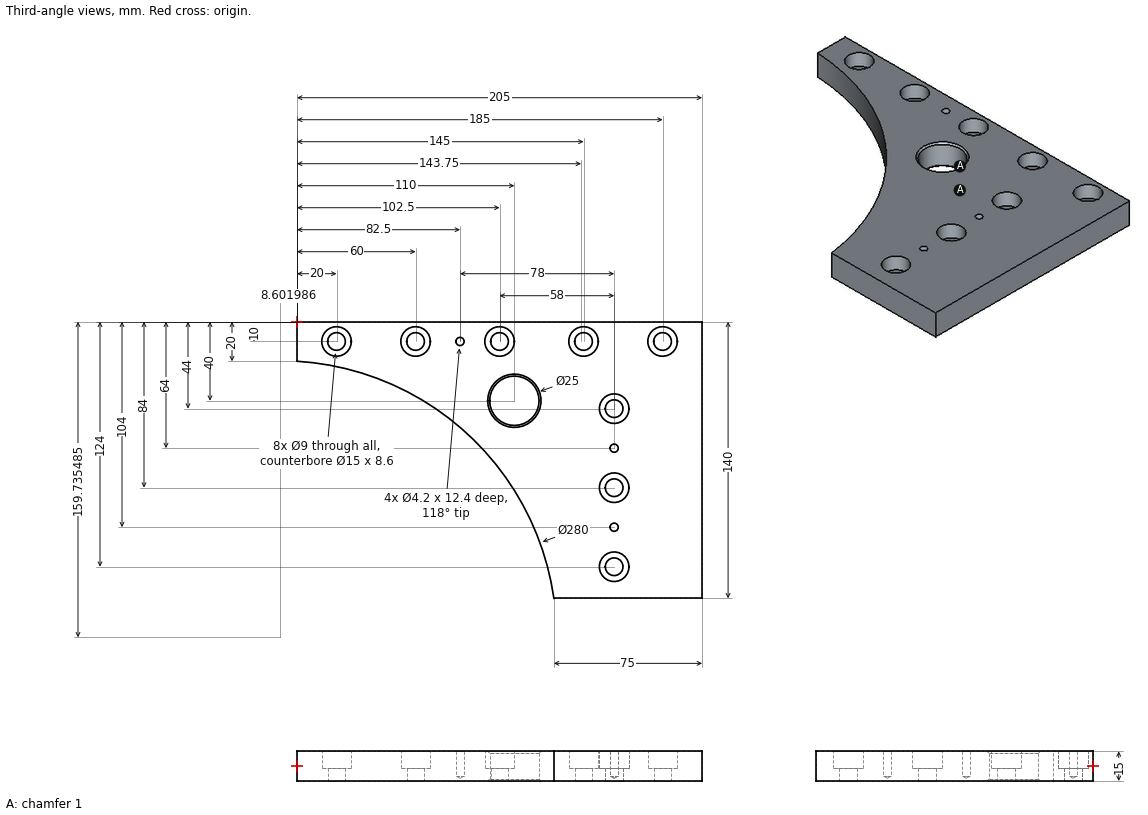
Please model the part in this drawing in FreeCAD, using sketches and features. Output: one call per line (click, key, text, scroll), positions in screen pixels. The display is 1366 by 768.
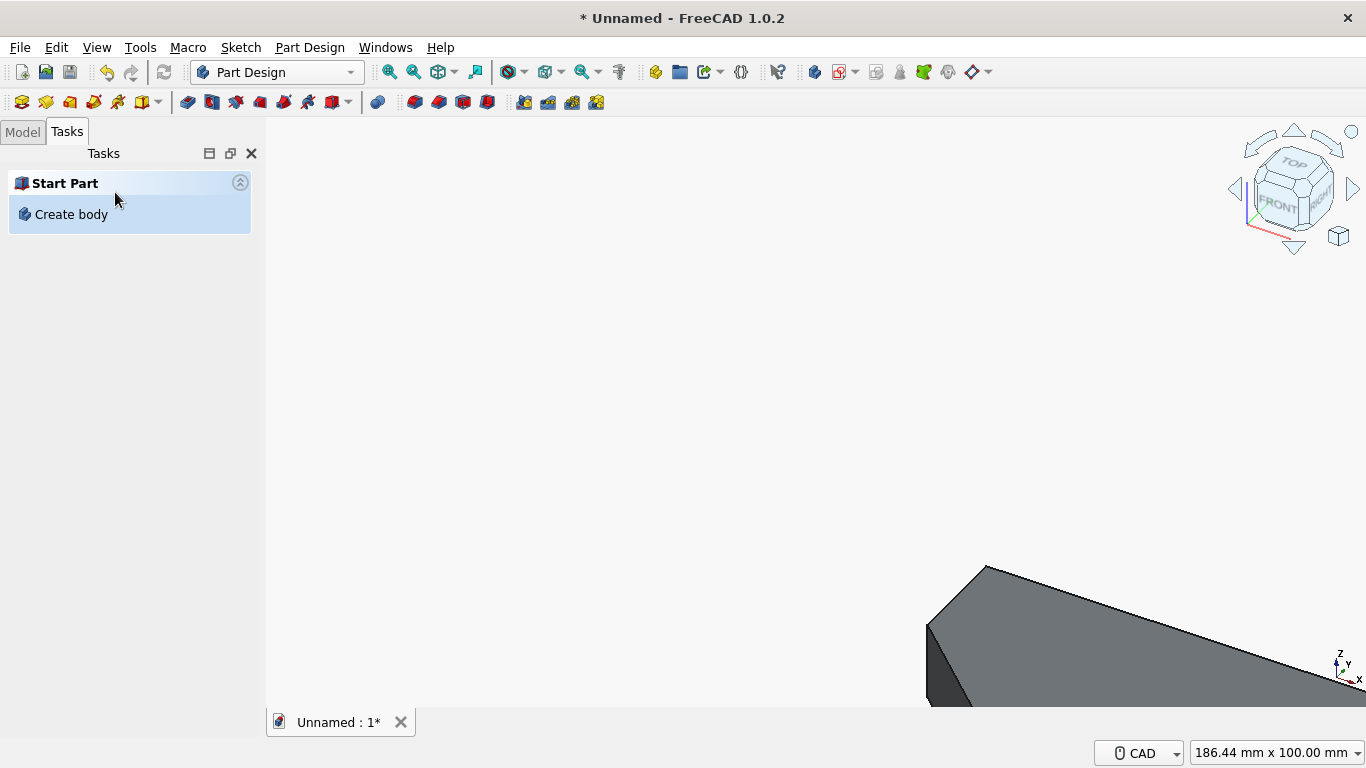
click(390, 72)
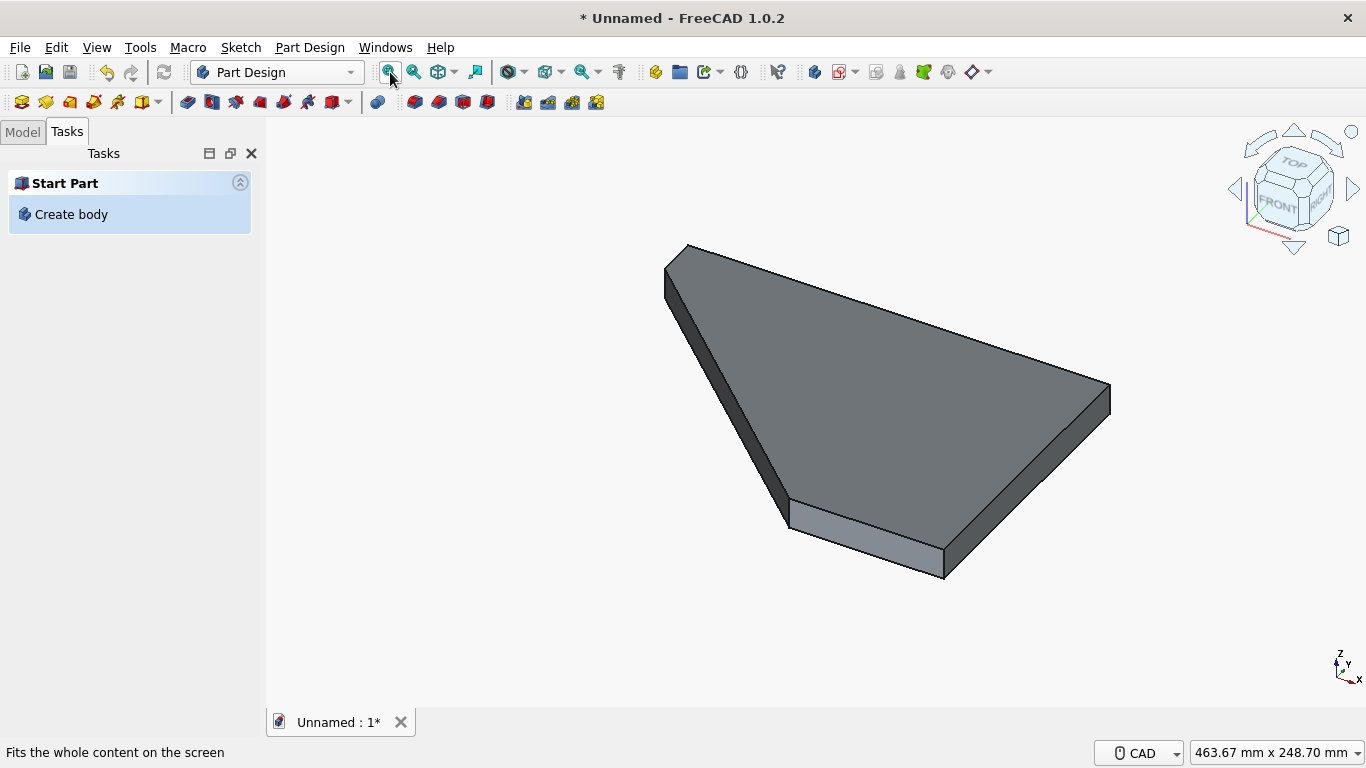
click(876, 416)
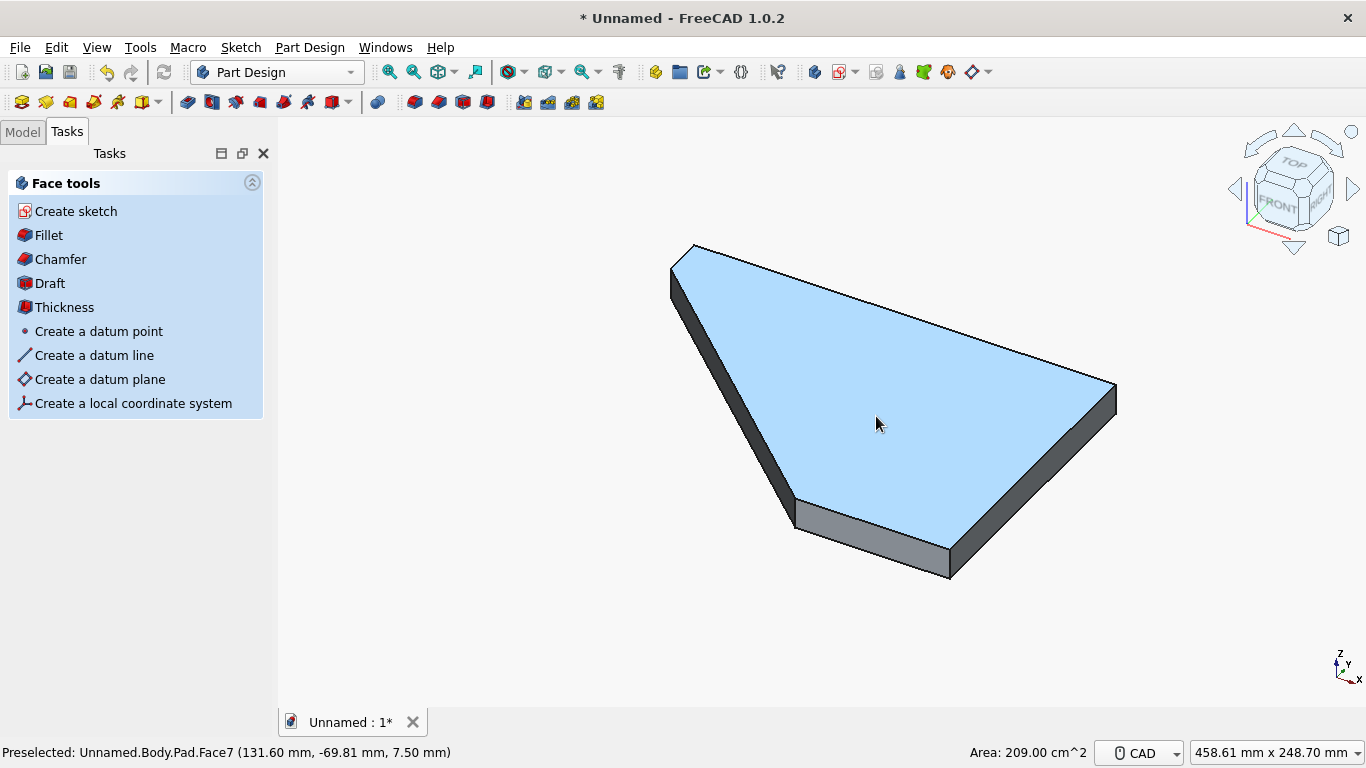
click(840, 72)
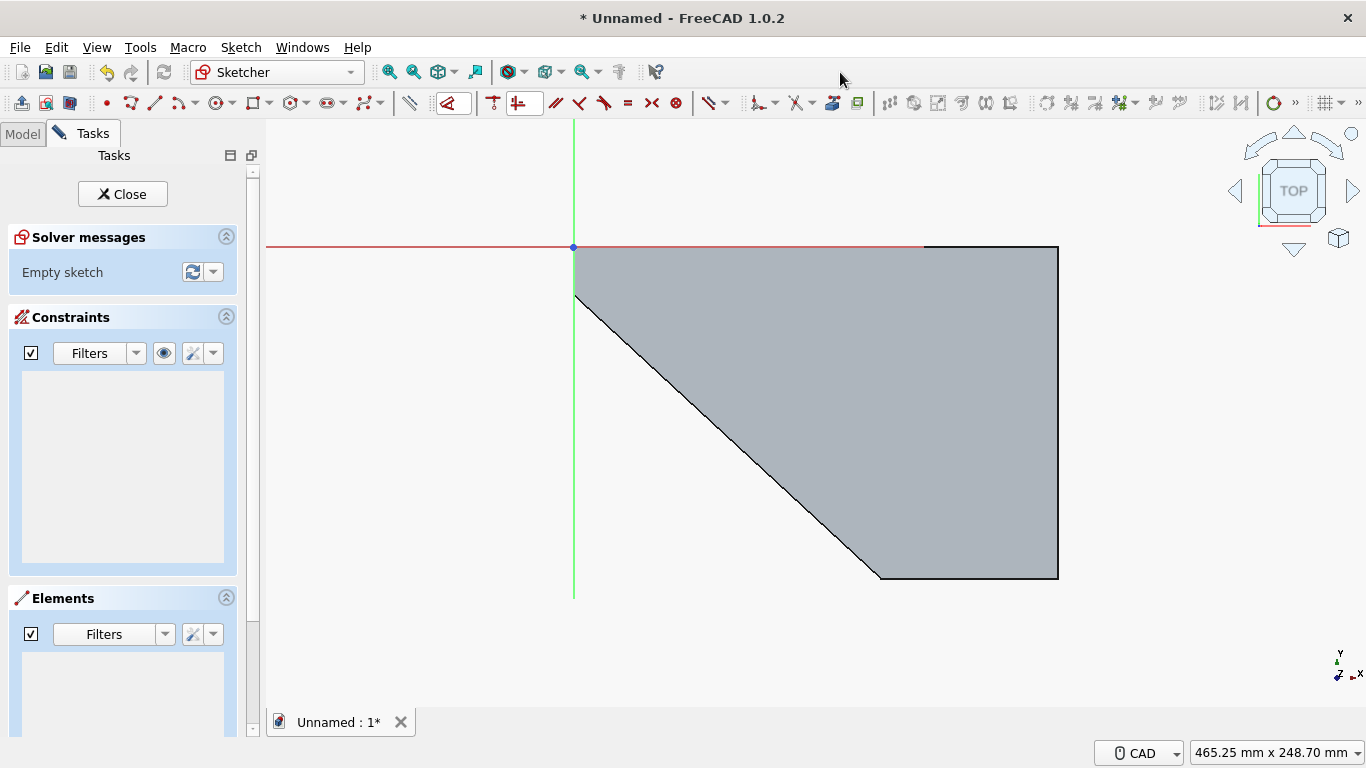
click(216, 104)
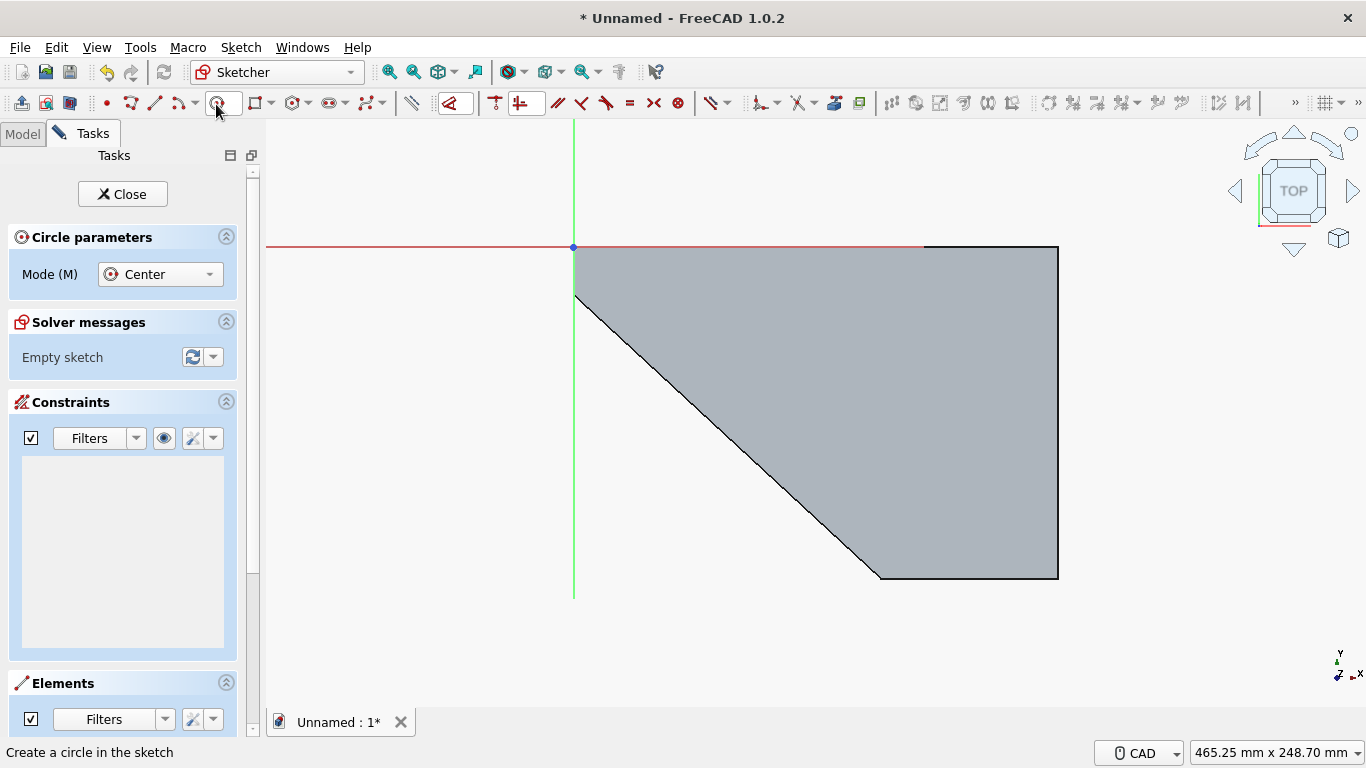
scroll(621, 271, up, 4)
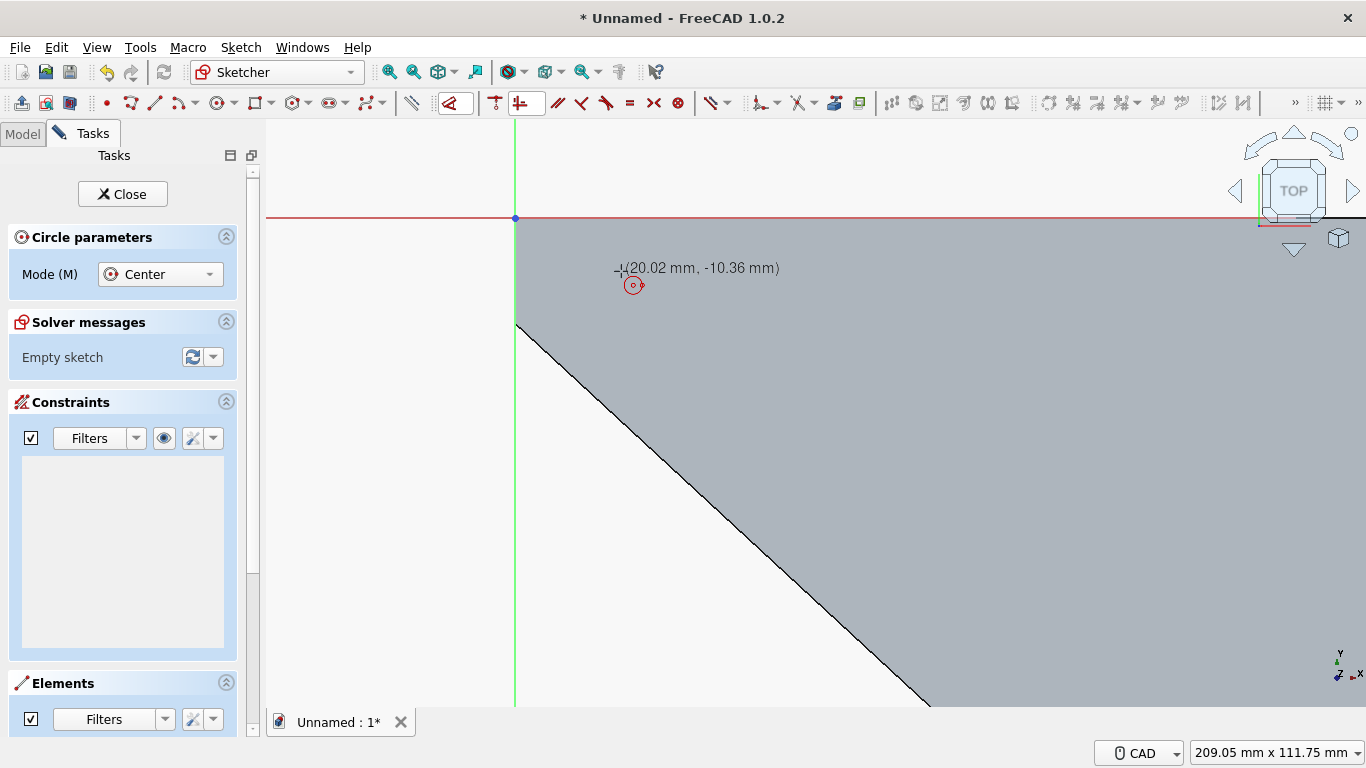
click(620, 271)
click(637, 254)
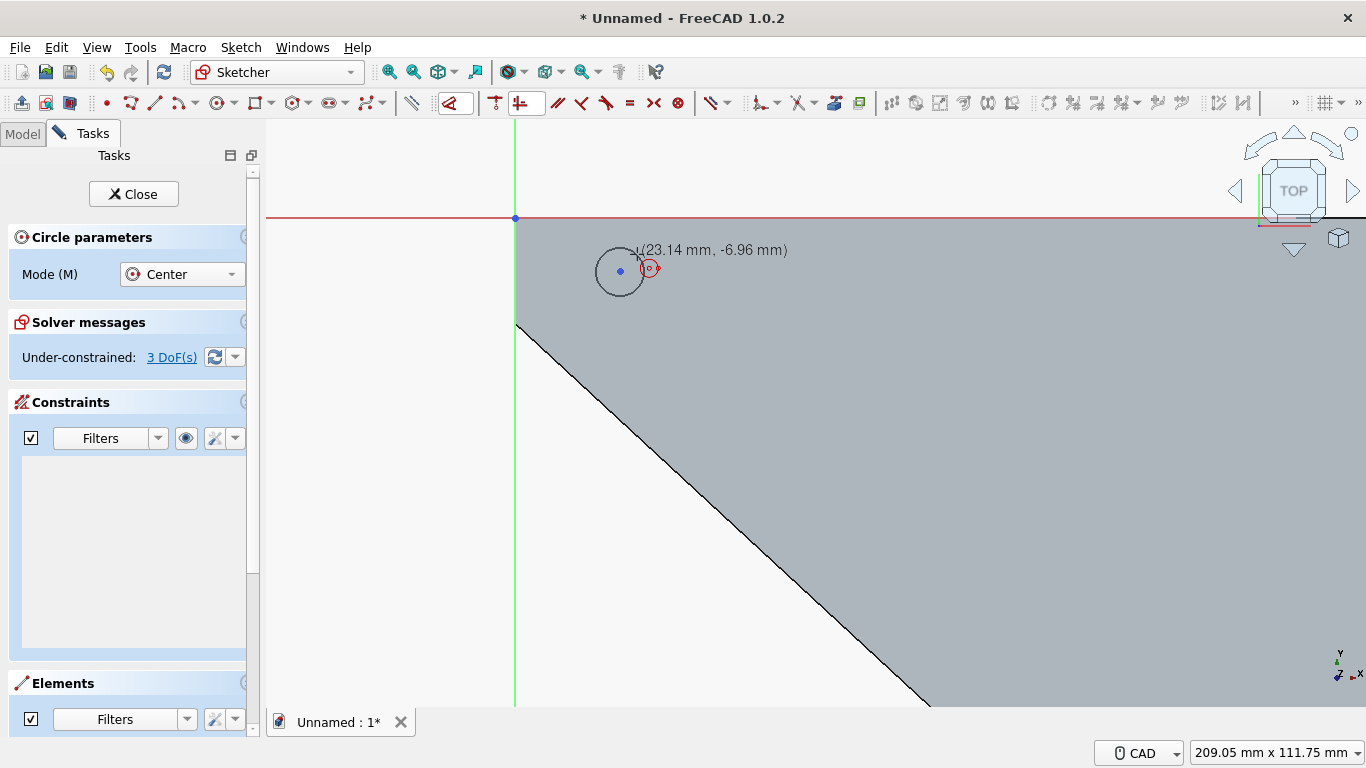
click(831, 271)
click(848, 254)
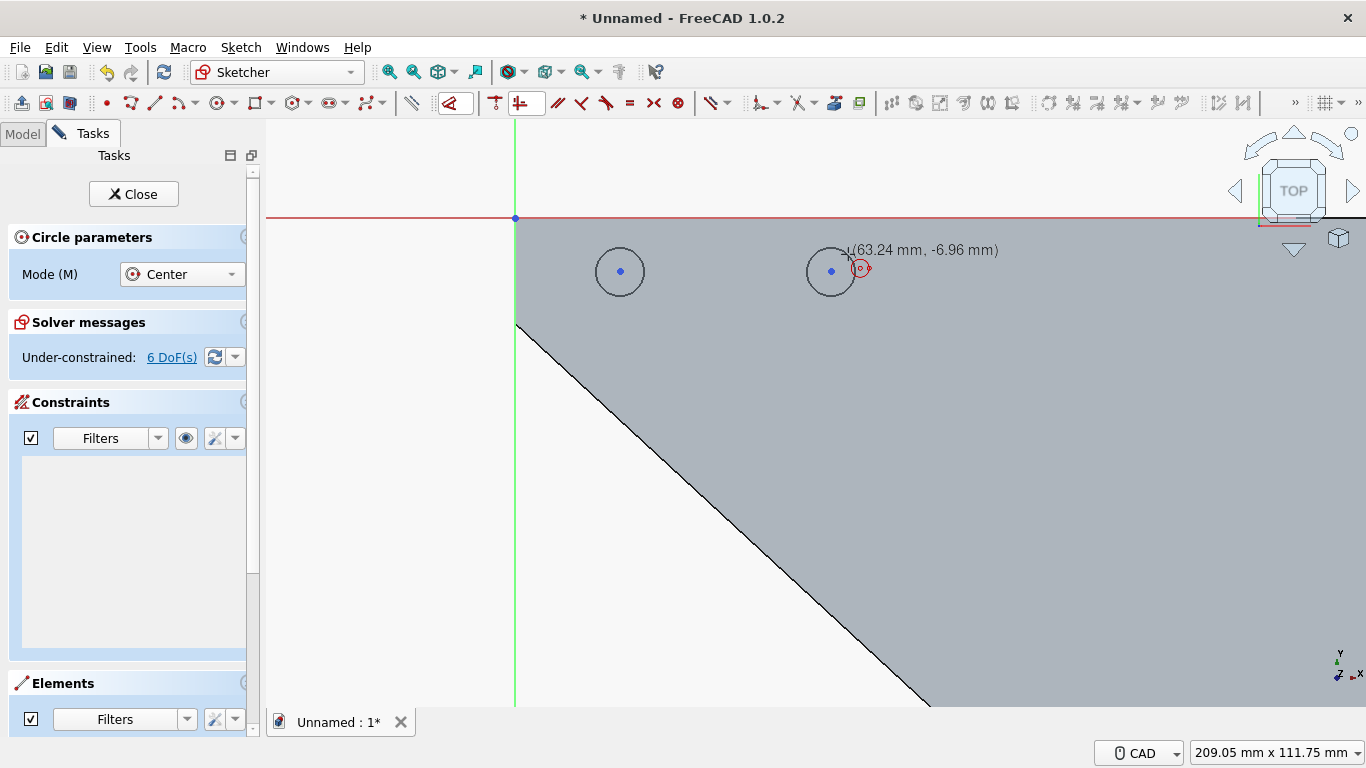
scroll(424, 239, down, 3)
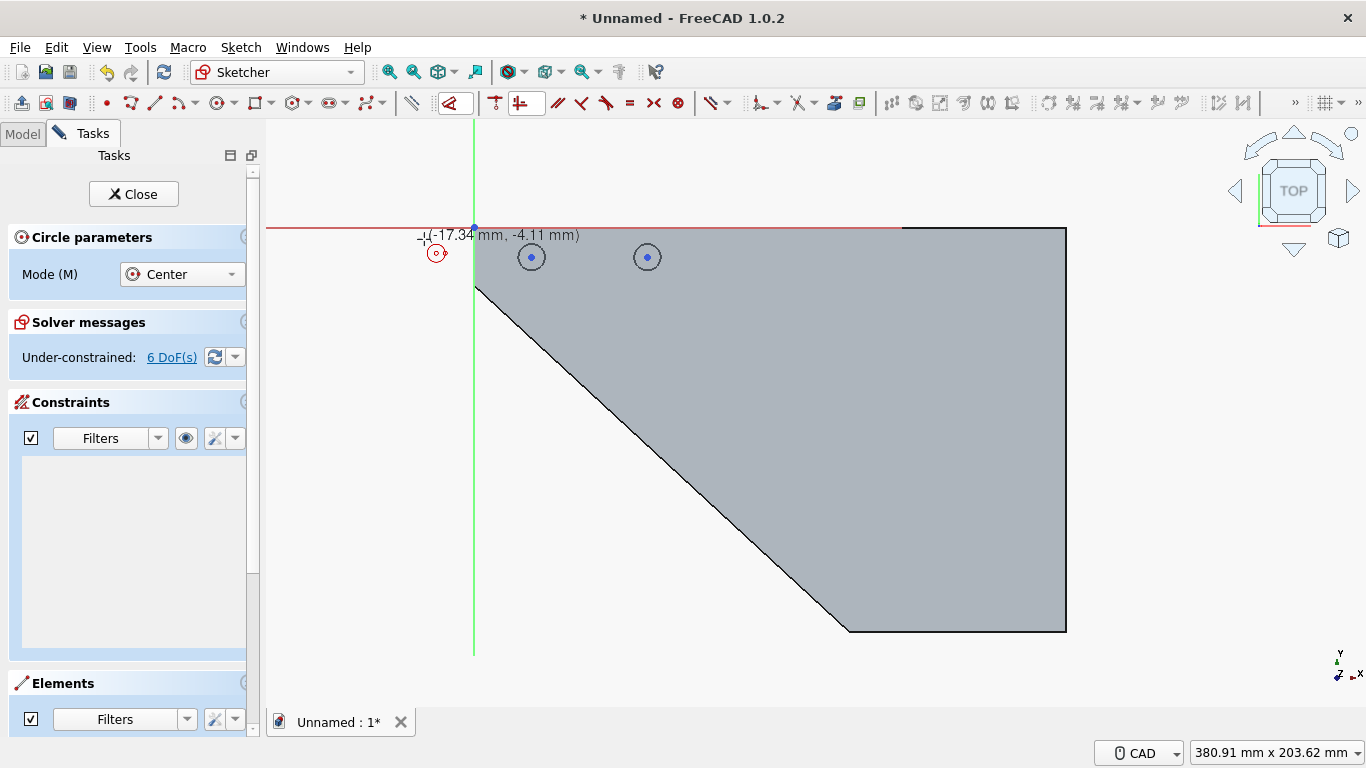
scroll(893, 257, up, 3)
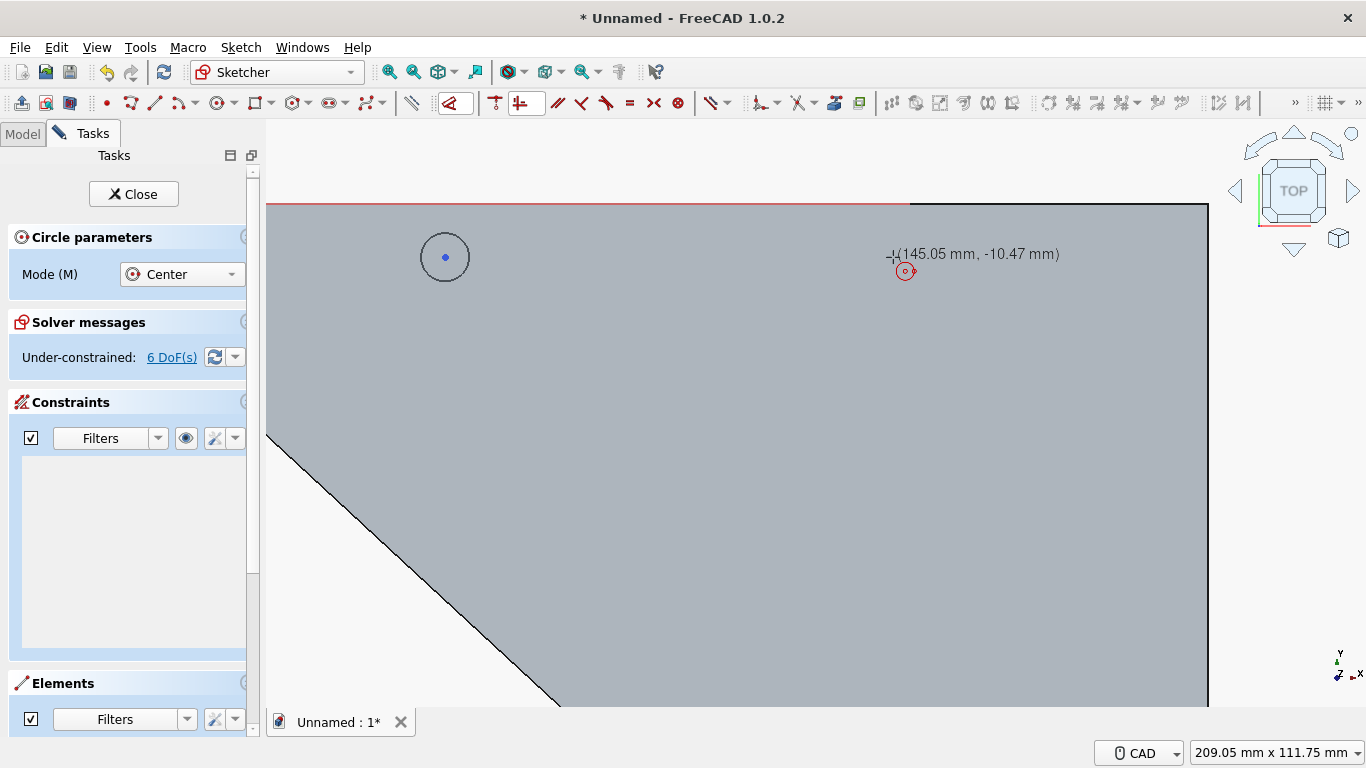
click(892, 256)
click(909, 239)